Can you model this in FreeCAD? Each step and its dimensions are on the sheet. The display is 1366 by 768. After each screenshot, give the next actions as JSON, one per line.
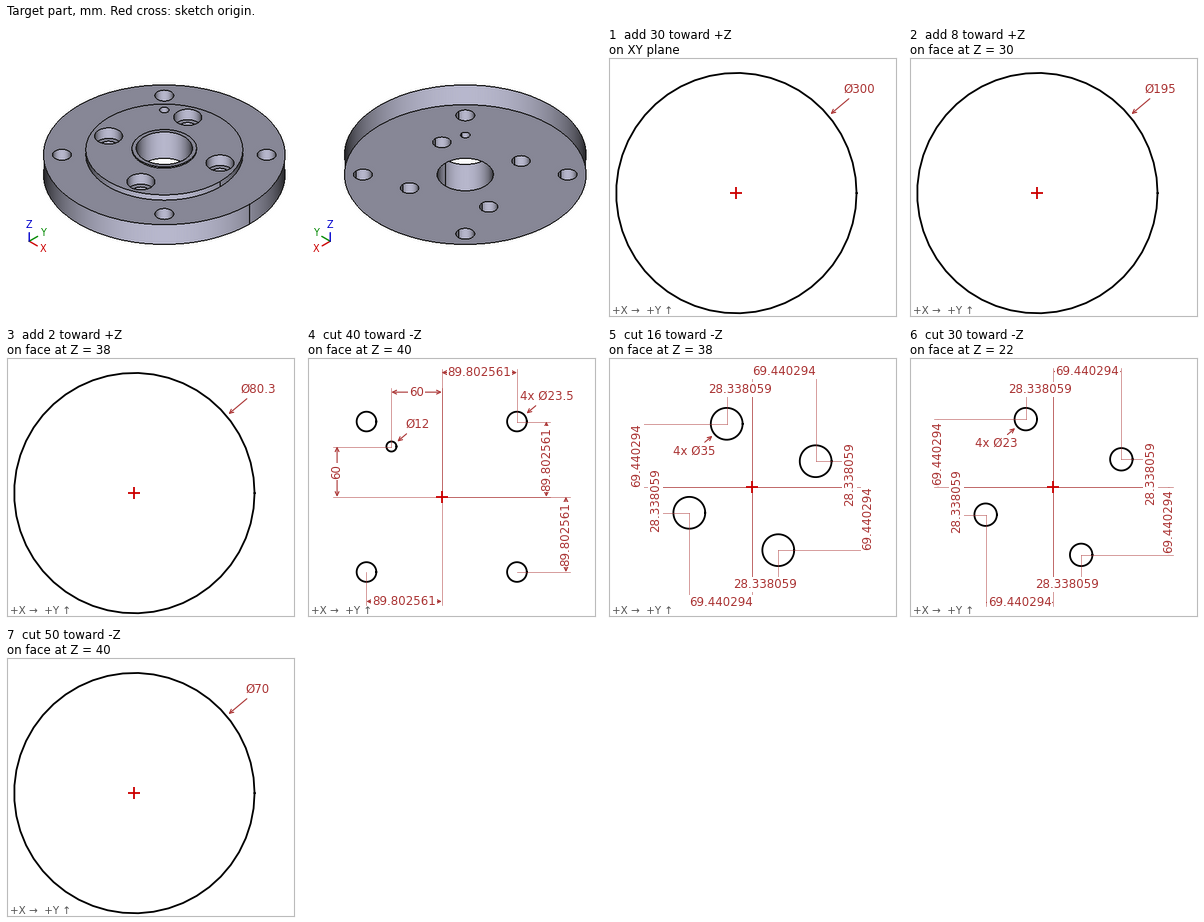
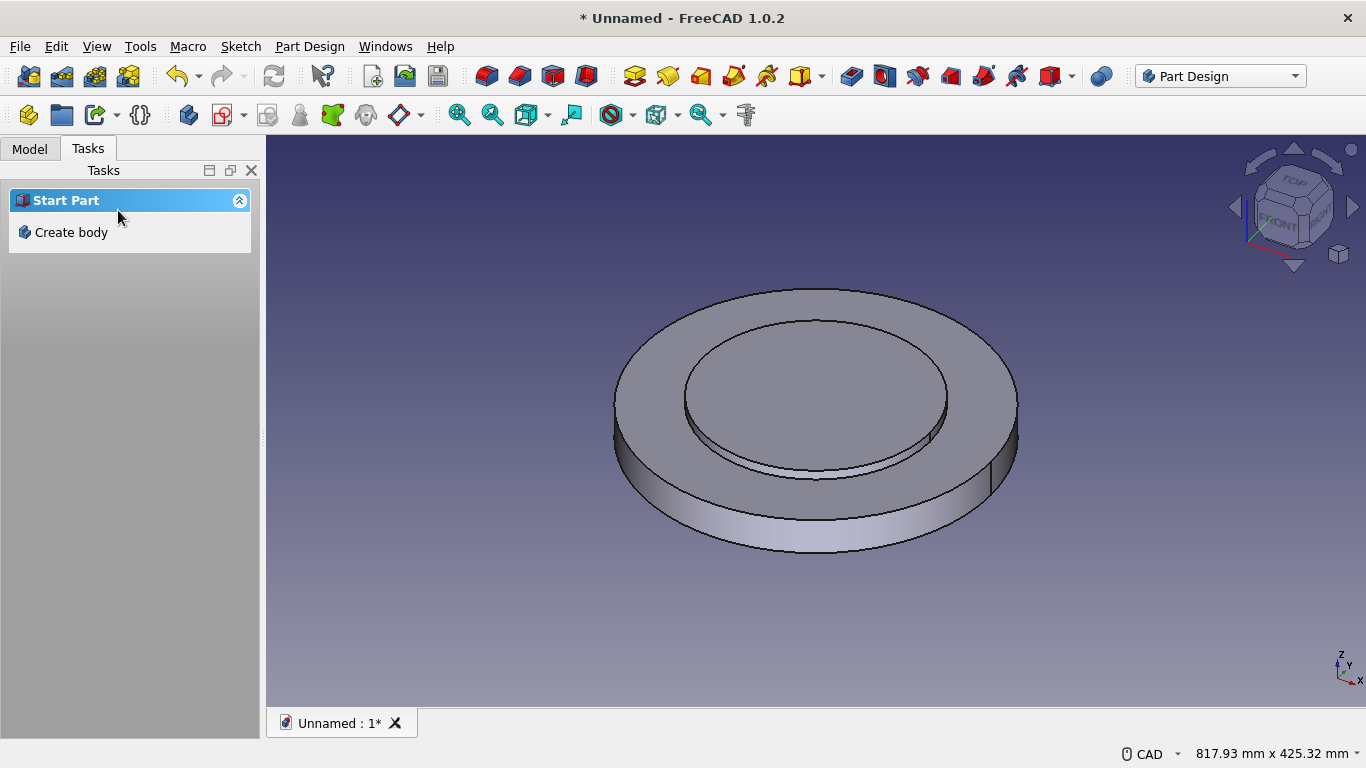
{"action": "left_click", "coordinate": [816, 395]}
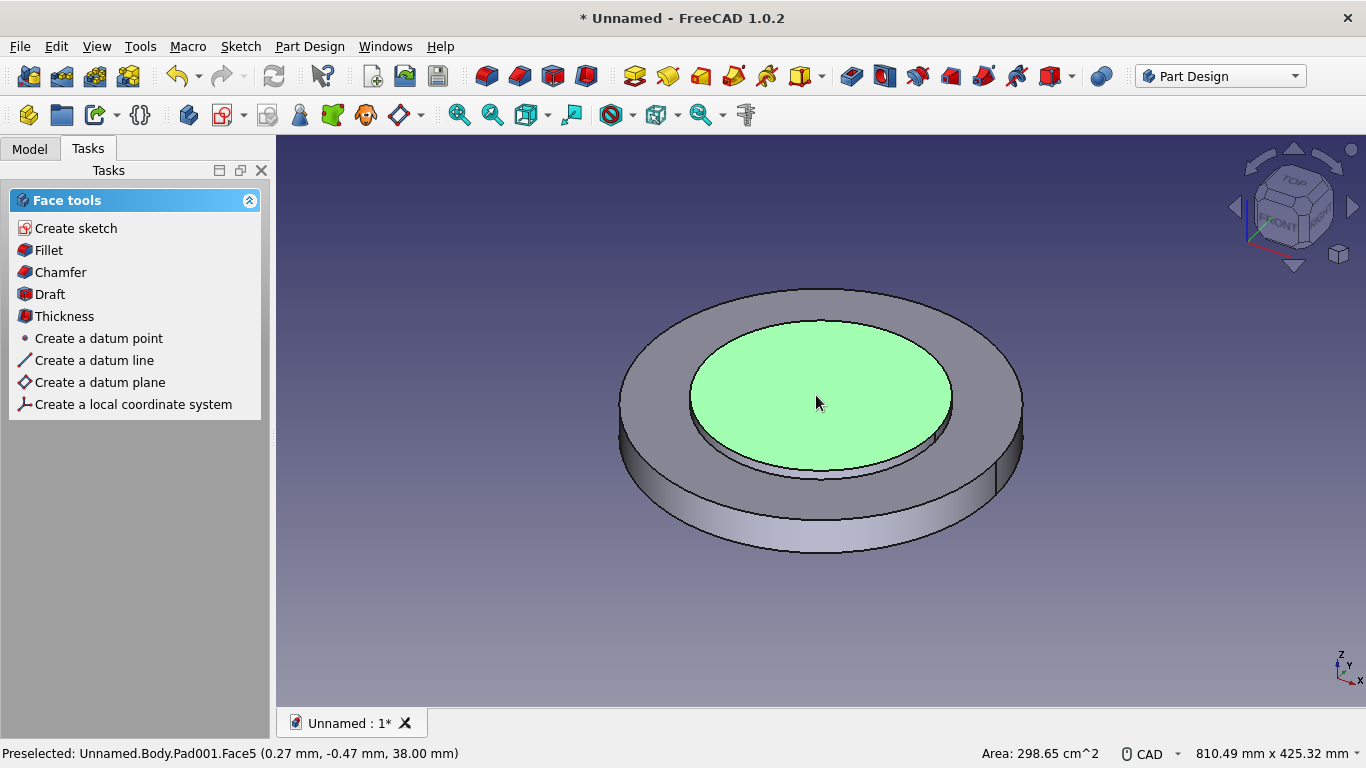
{"action": "left_click", "coordinate": [222, 116]}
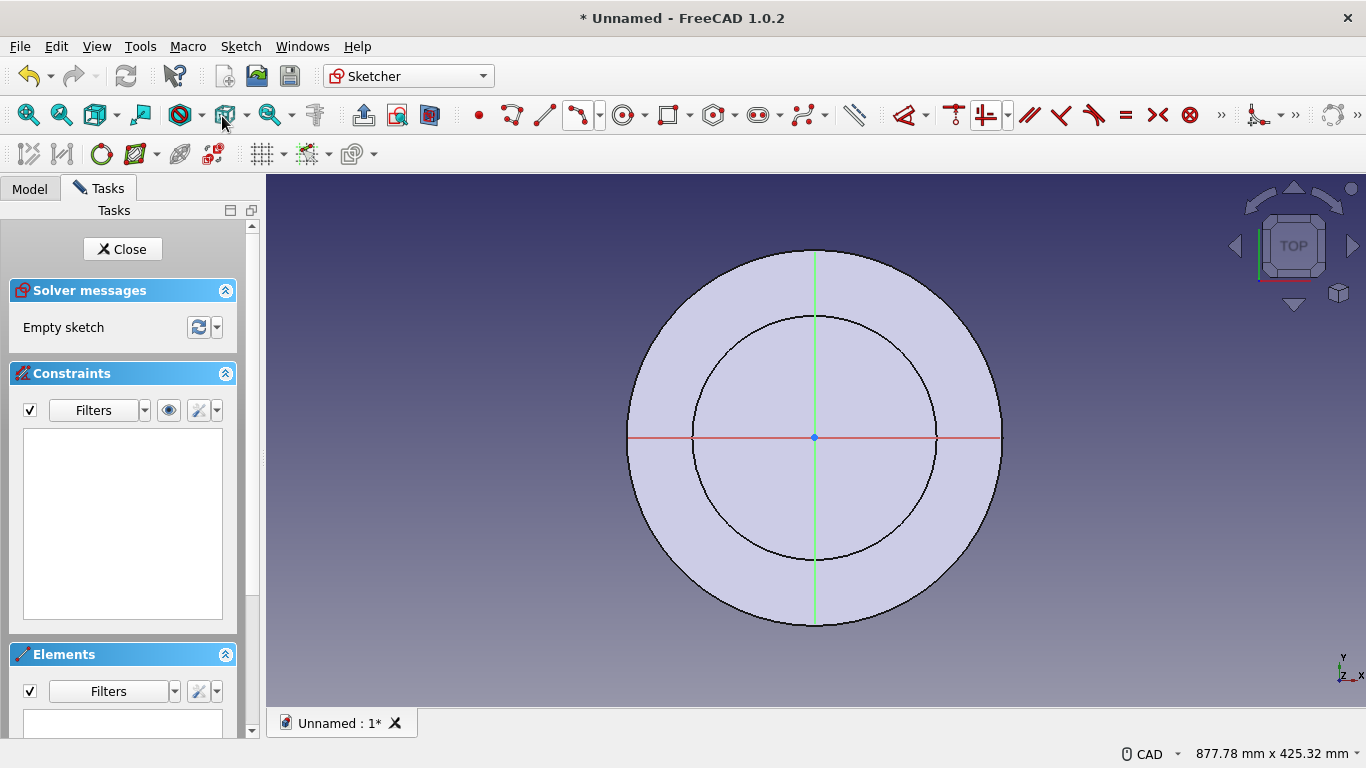
{"action": "scroll", "coordinate": [843, 437], "scroll_direction": "up", "scroll_amount": 6}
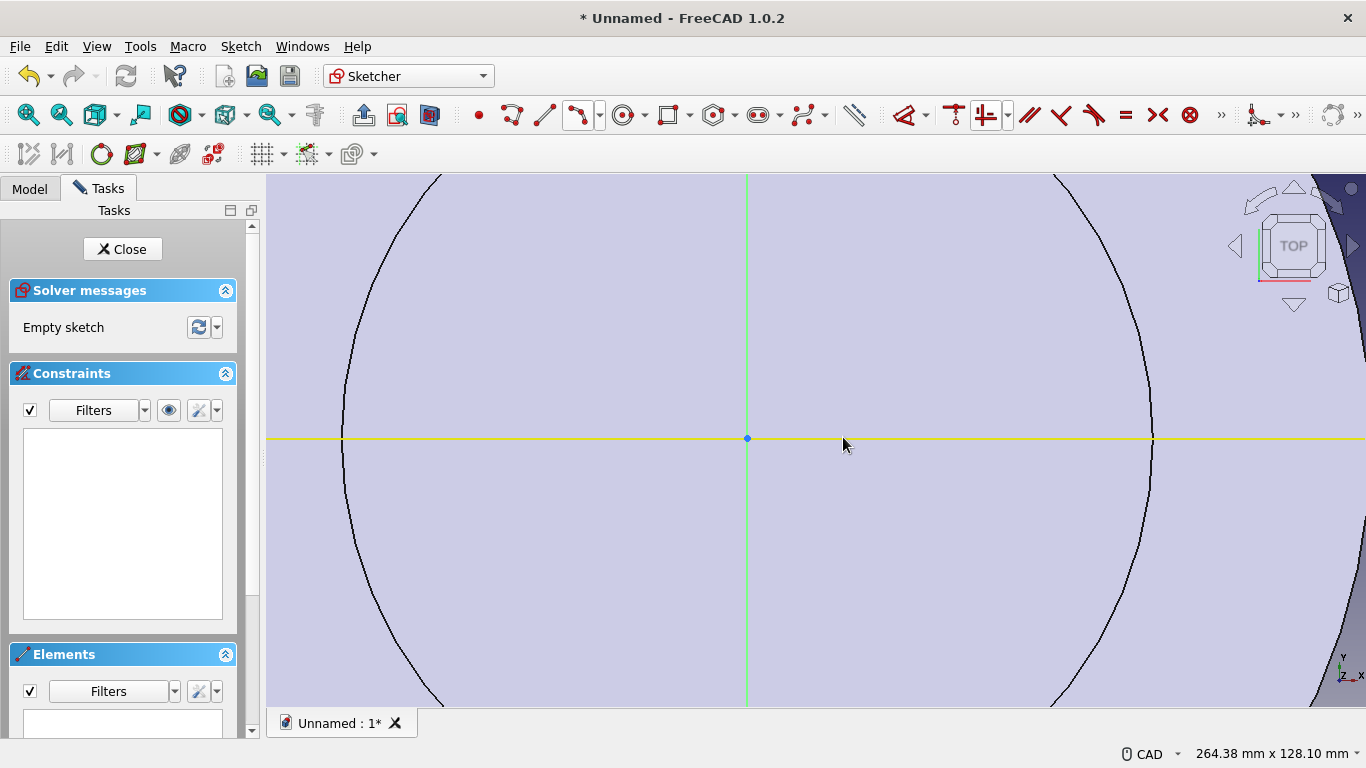
{"action": "left_click", "coordinate": [622, 116]}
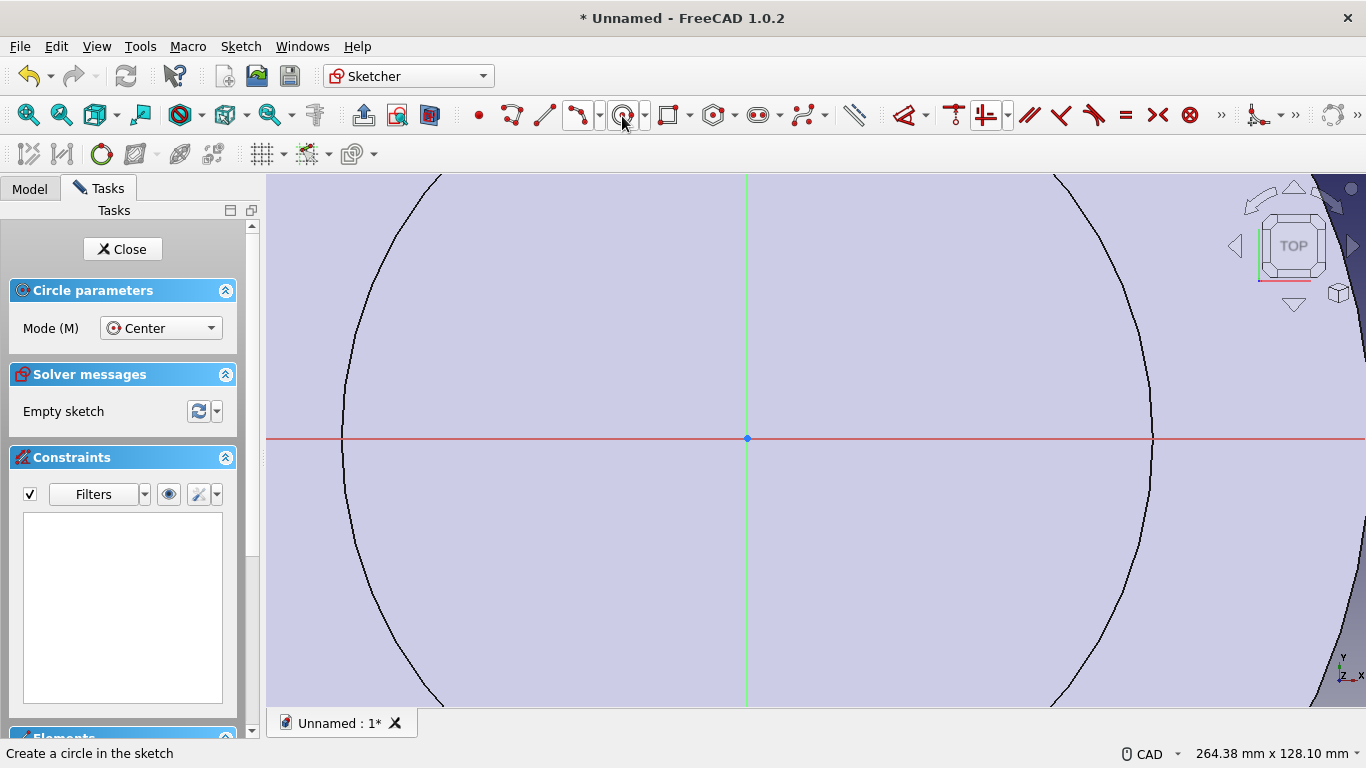
{"action": "left_click", "coordinate": [747, 439]}
{"action": "left_click", "coordinate": [865, 321]}
{"action": "key", "text": "Escape"}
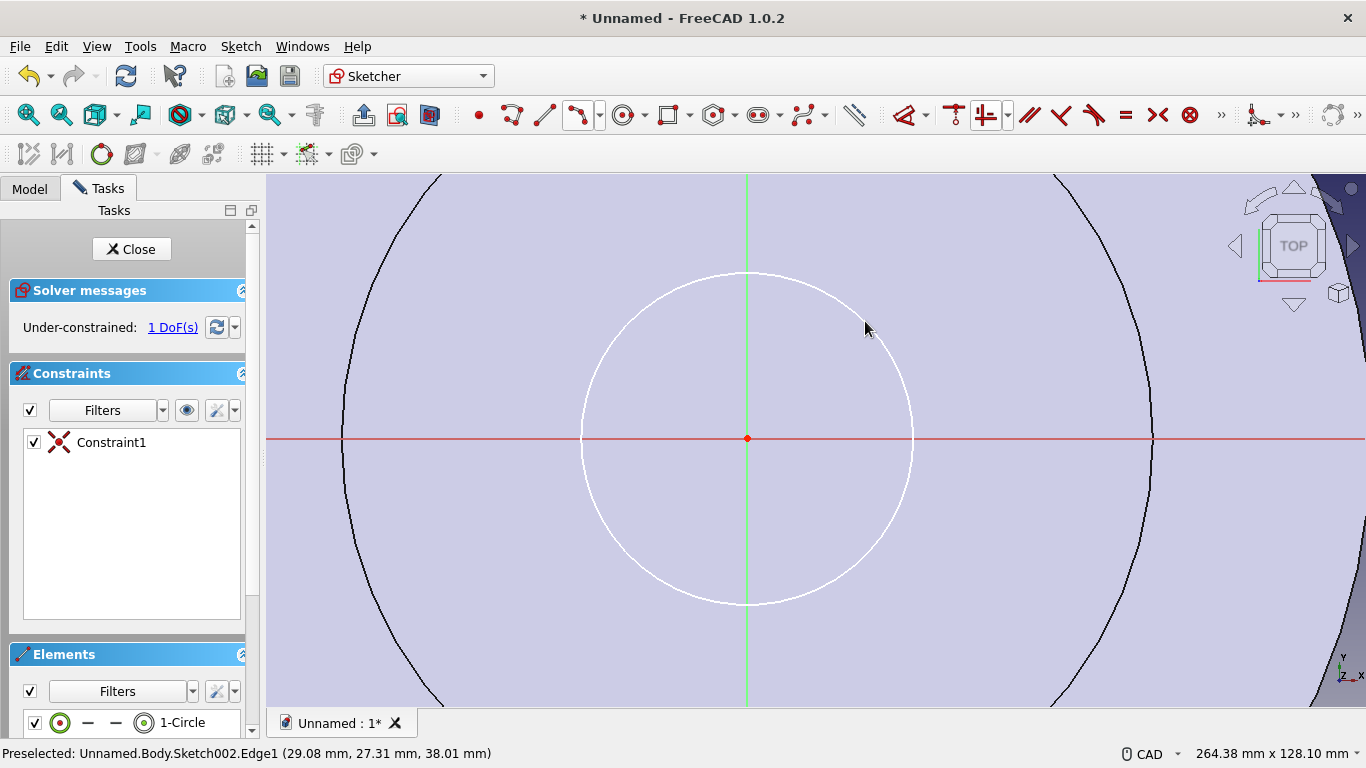
{"action": "left_click", "coordinate": [904, 116]}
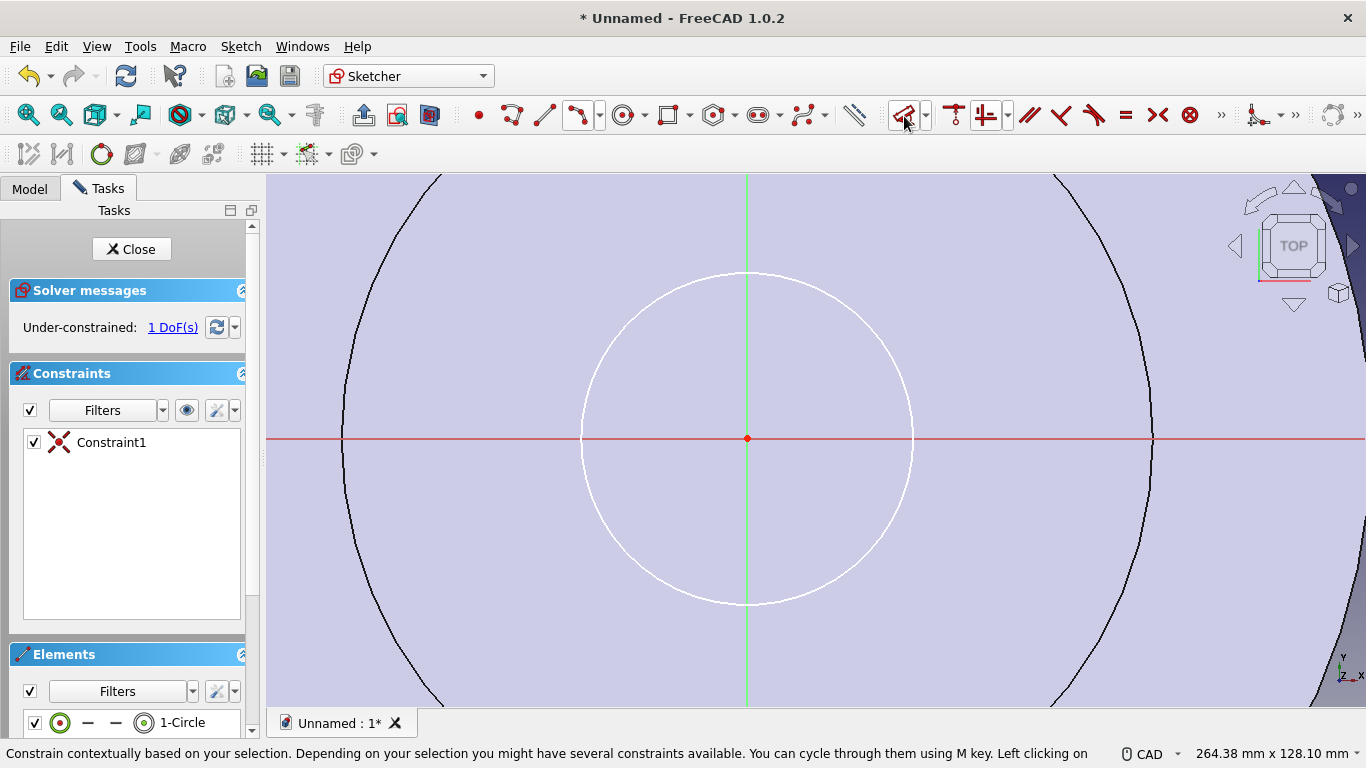
{"action": "left_click", "coordinate": [864, 321]}
{"action": "left_click", "coordinate": [887, 298]}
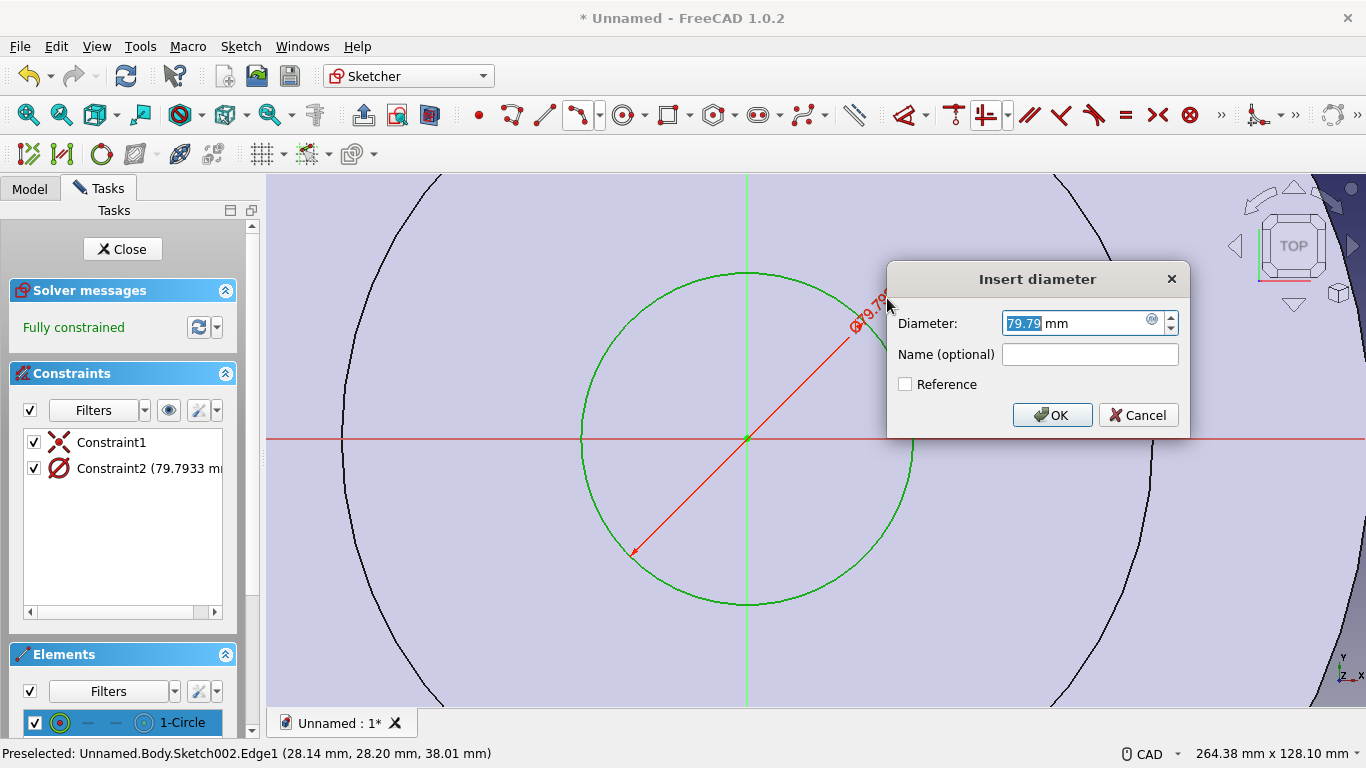
{"action": "type", "text": "80.3"}
{"action": "key", "text": "Return"}
{"action": "key", "text": "Escape"}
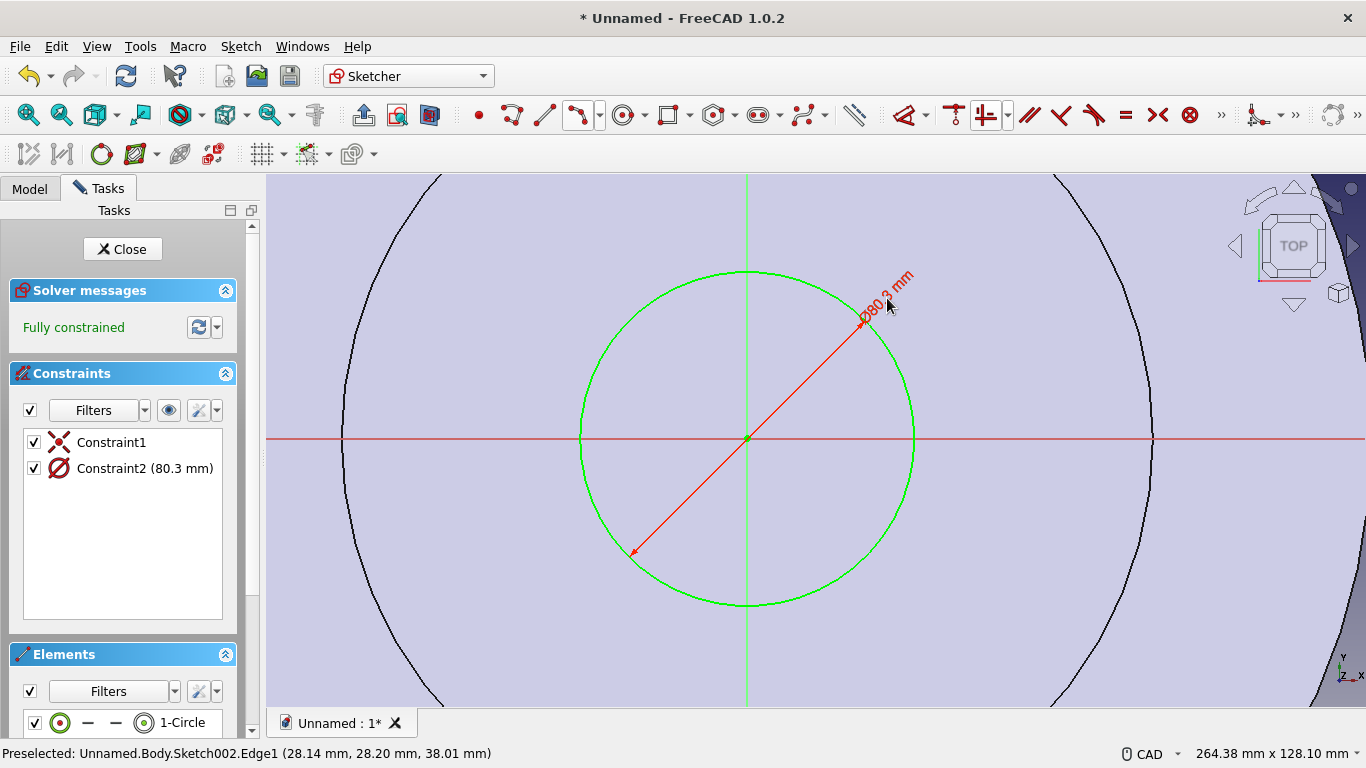
{"action": "left_click", "coordinate": [123, 249]}